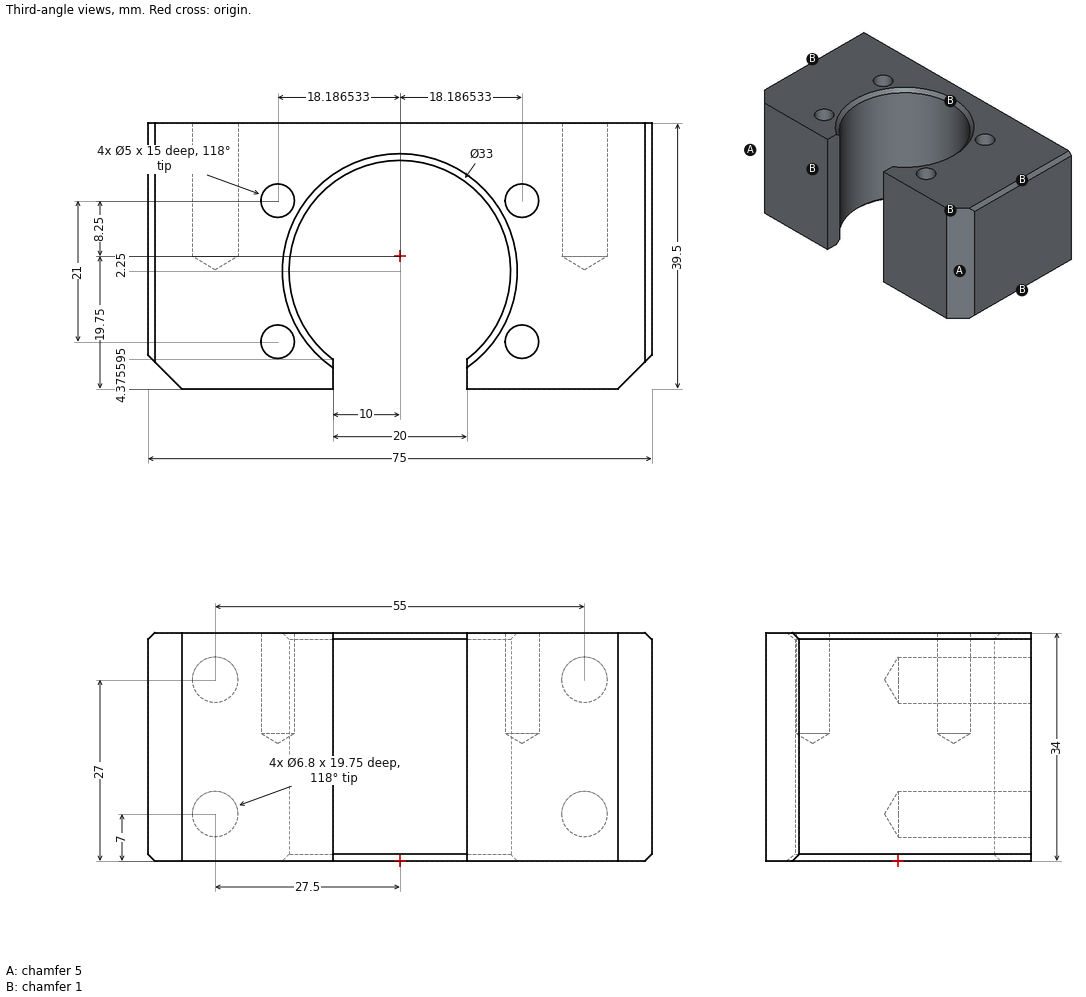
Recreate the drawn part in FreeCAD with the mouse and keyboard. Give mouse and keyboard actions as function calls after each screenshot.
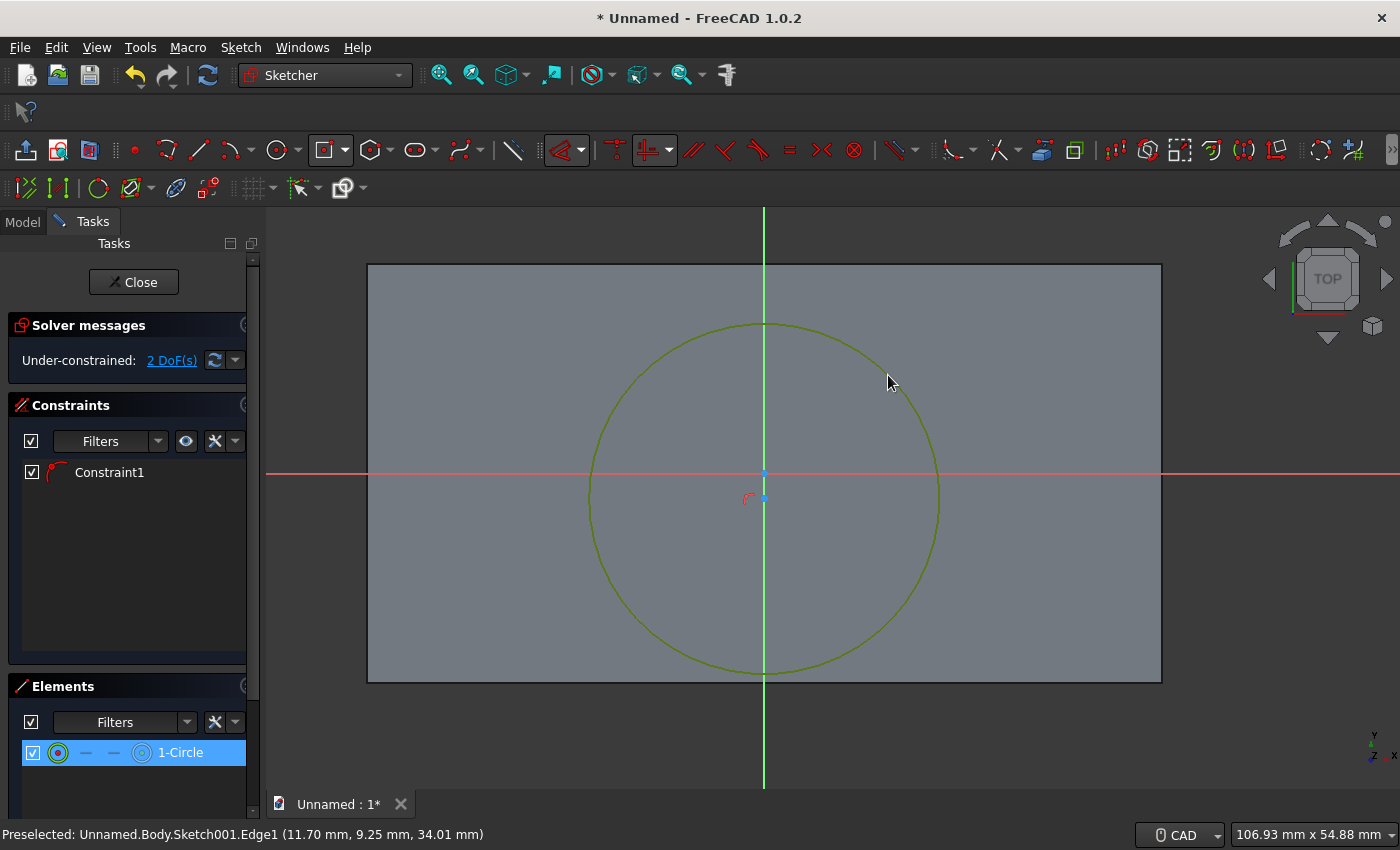
click(584, 150)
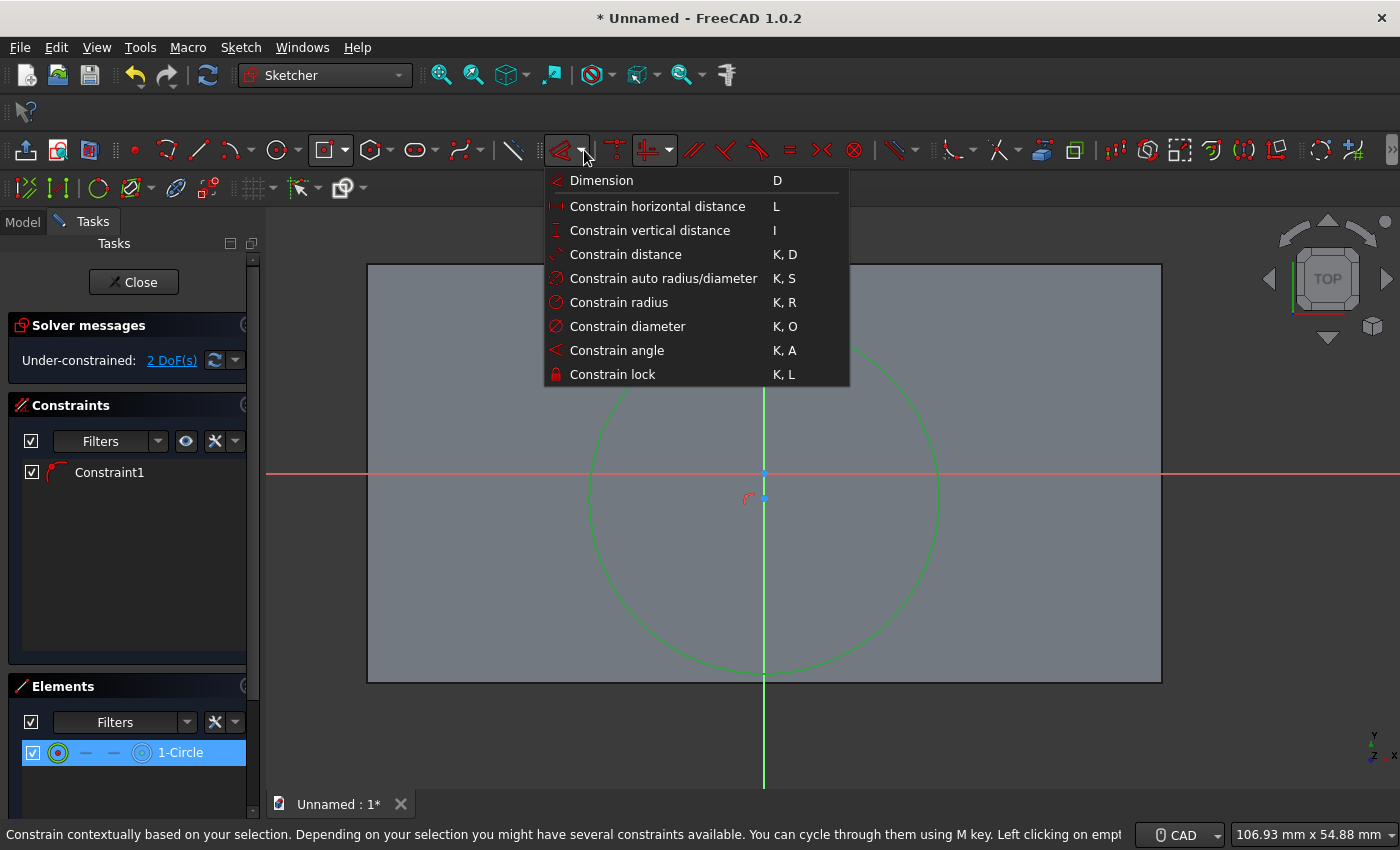
click(697, 326)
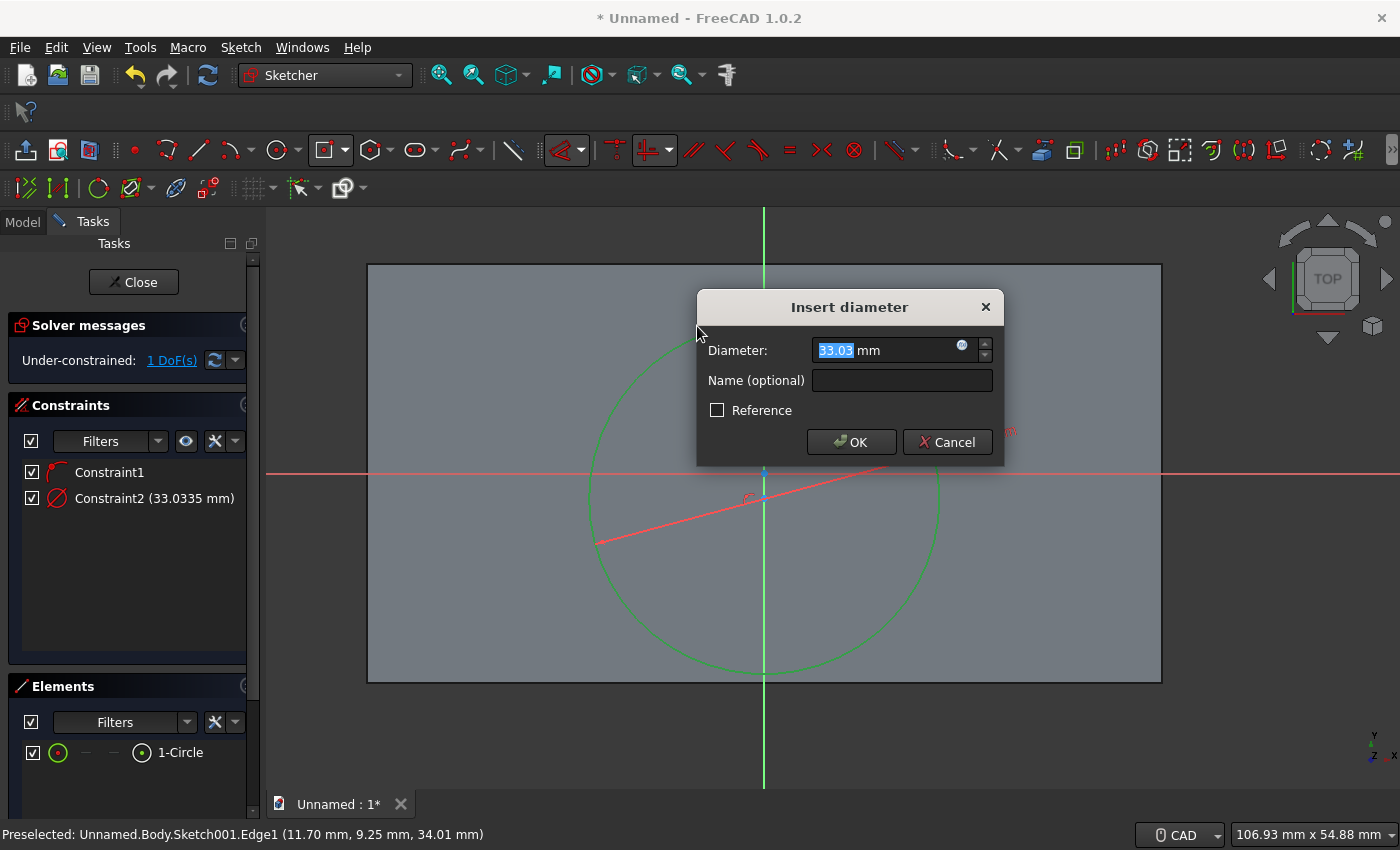
text(33)
key(Return)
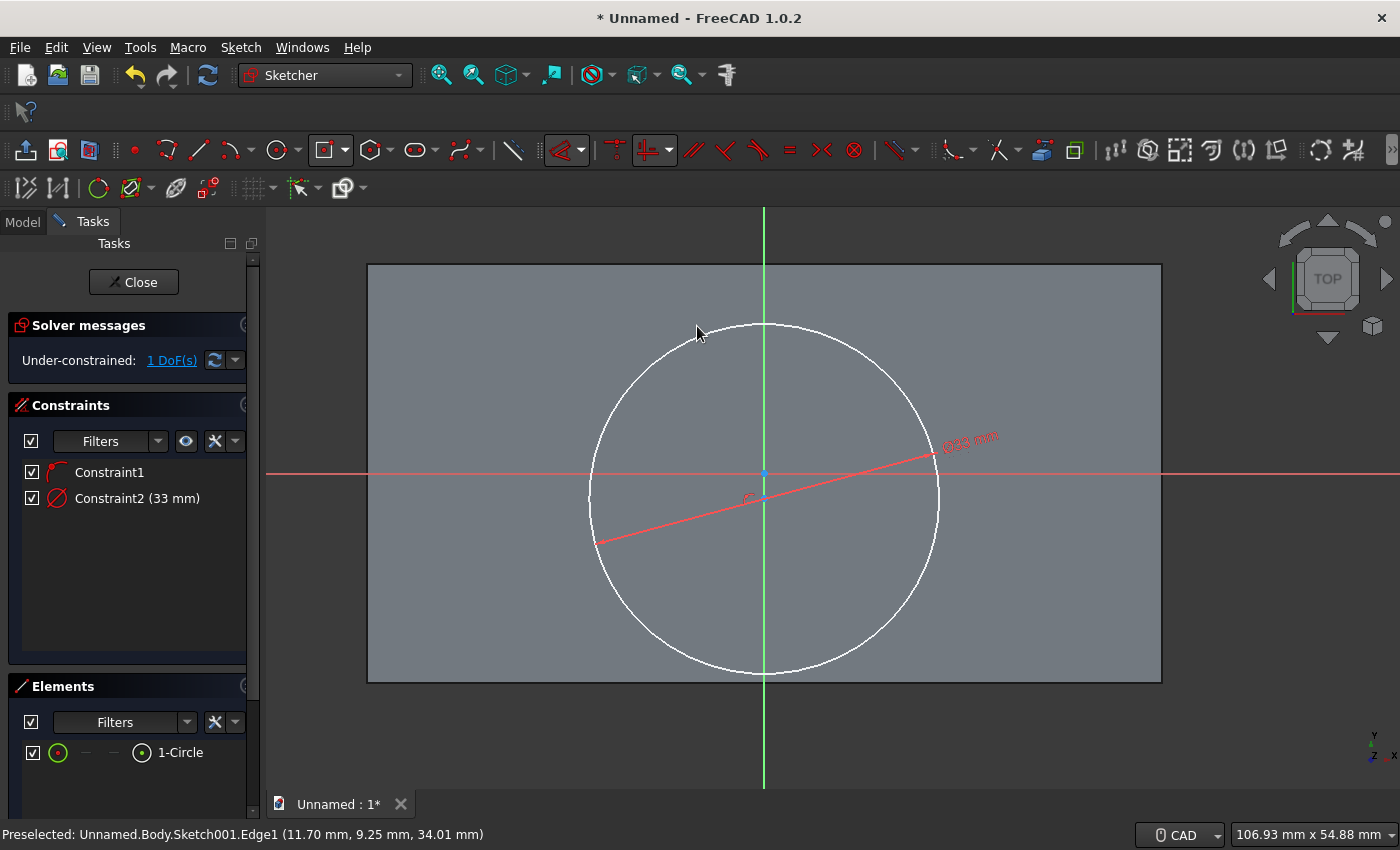
scroll(764, 499, up, 3)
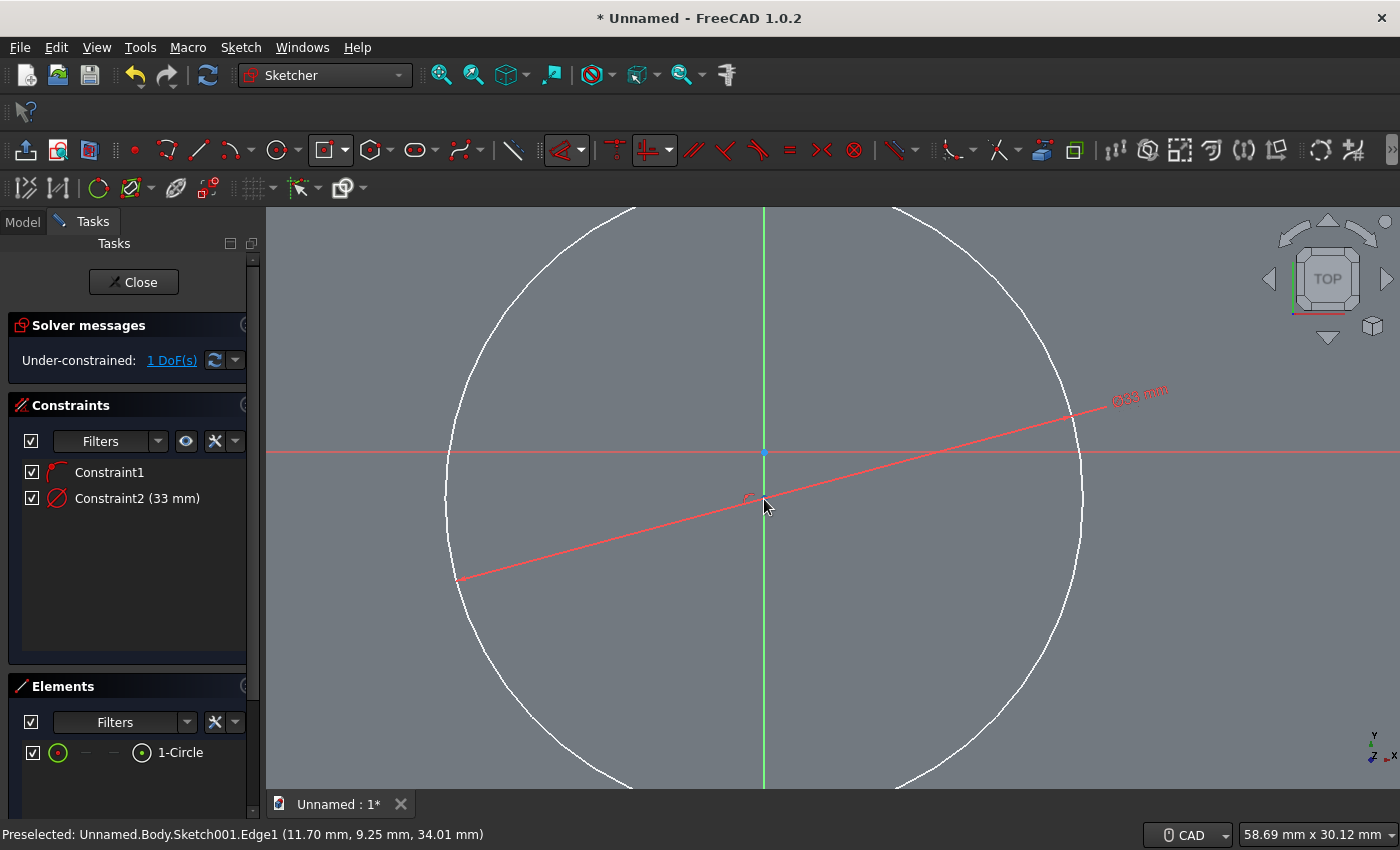
click(764, 499)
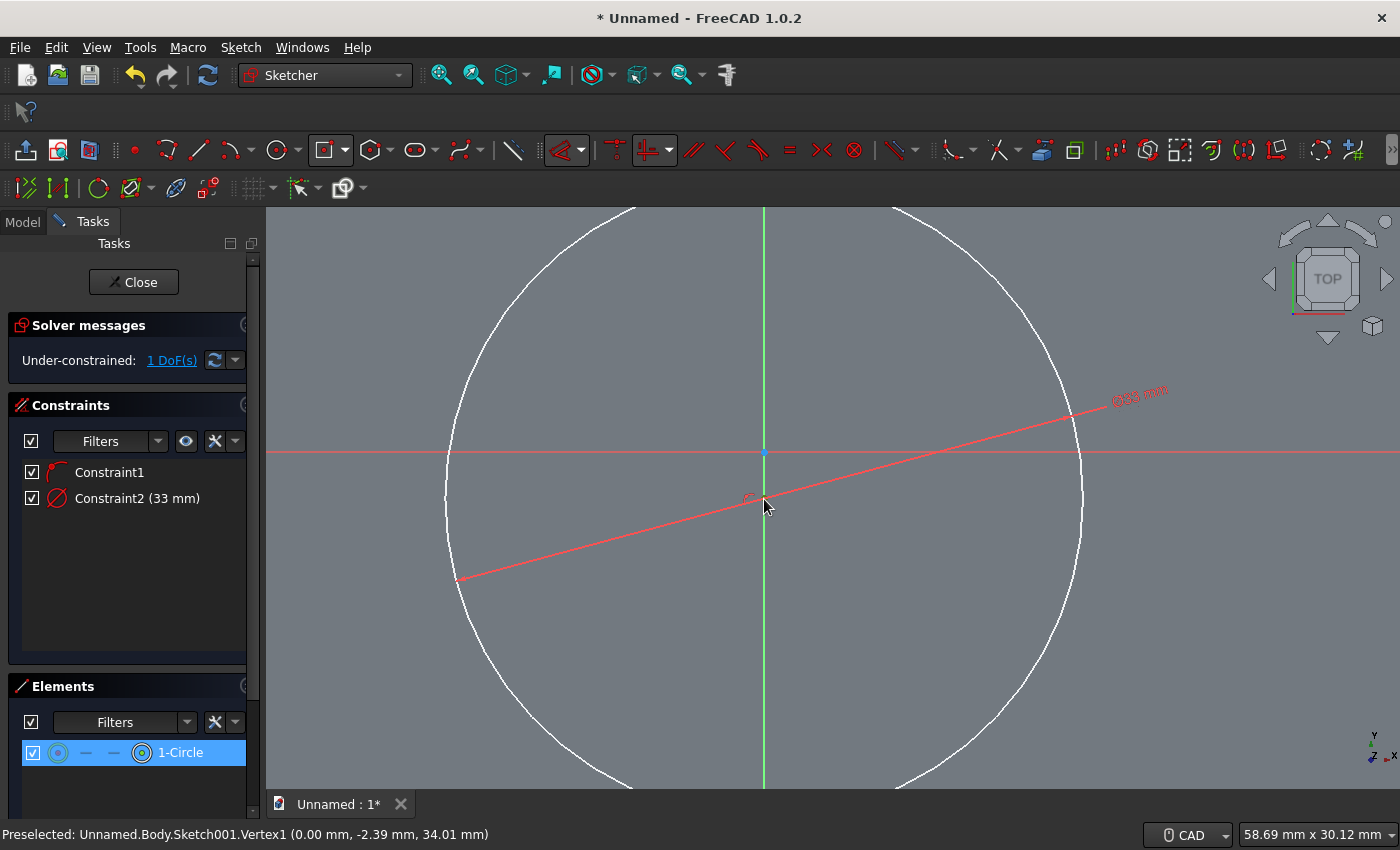
key(i)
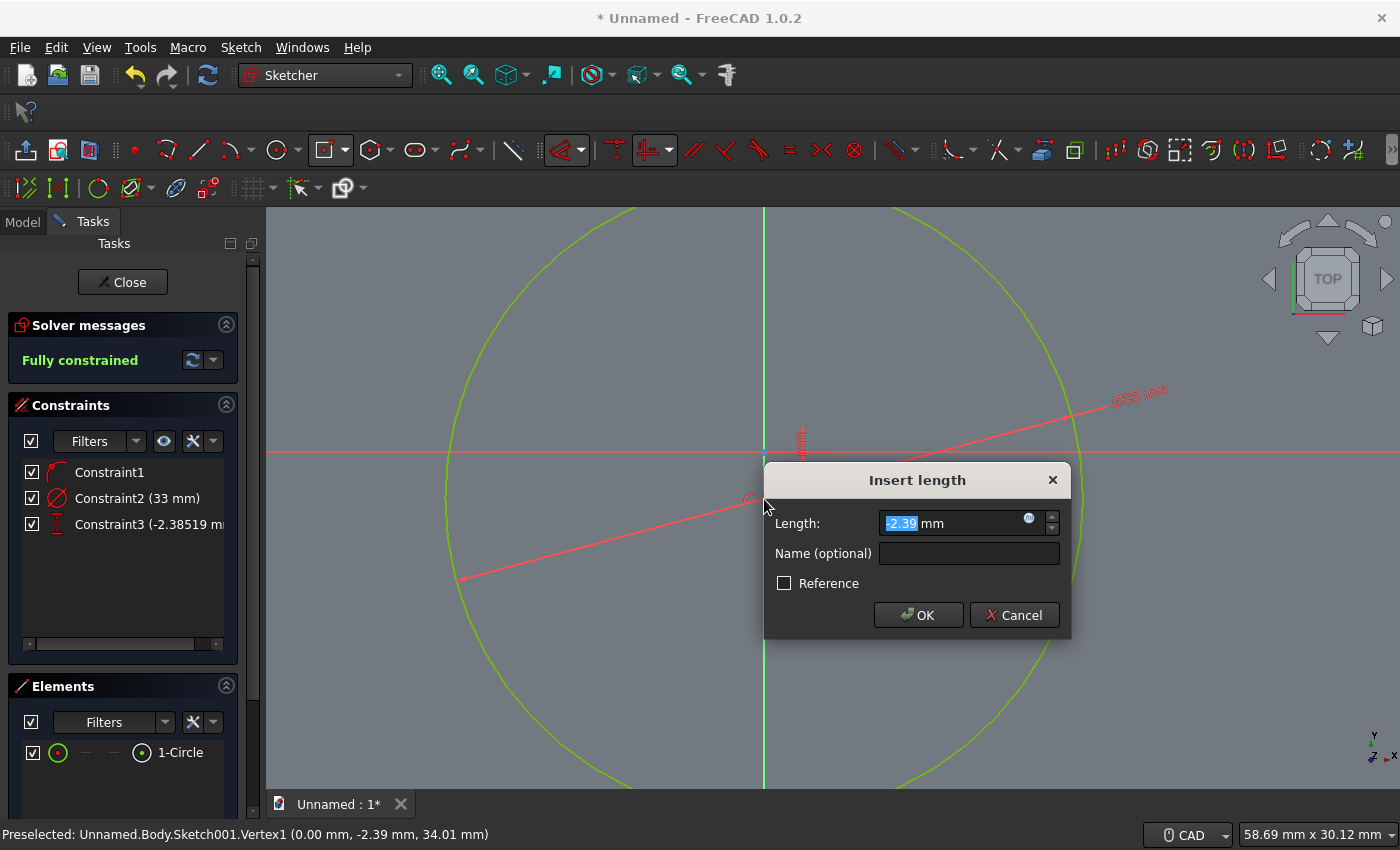
text(-2.25)
key(Return)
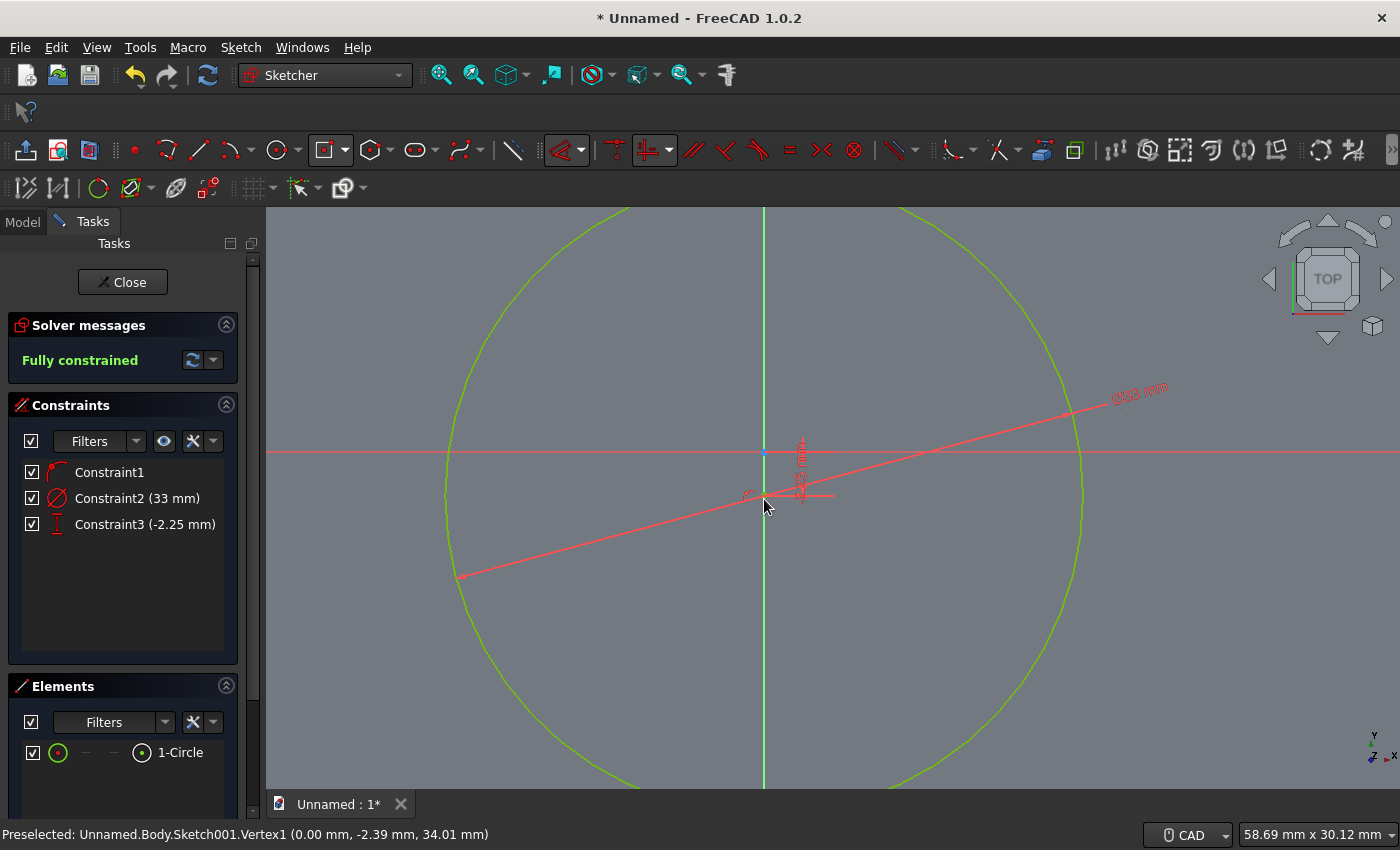
click(123, 282)